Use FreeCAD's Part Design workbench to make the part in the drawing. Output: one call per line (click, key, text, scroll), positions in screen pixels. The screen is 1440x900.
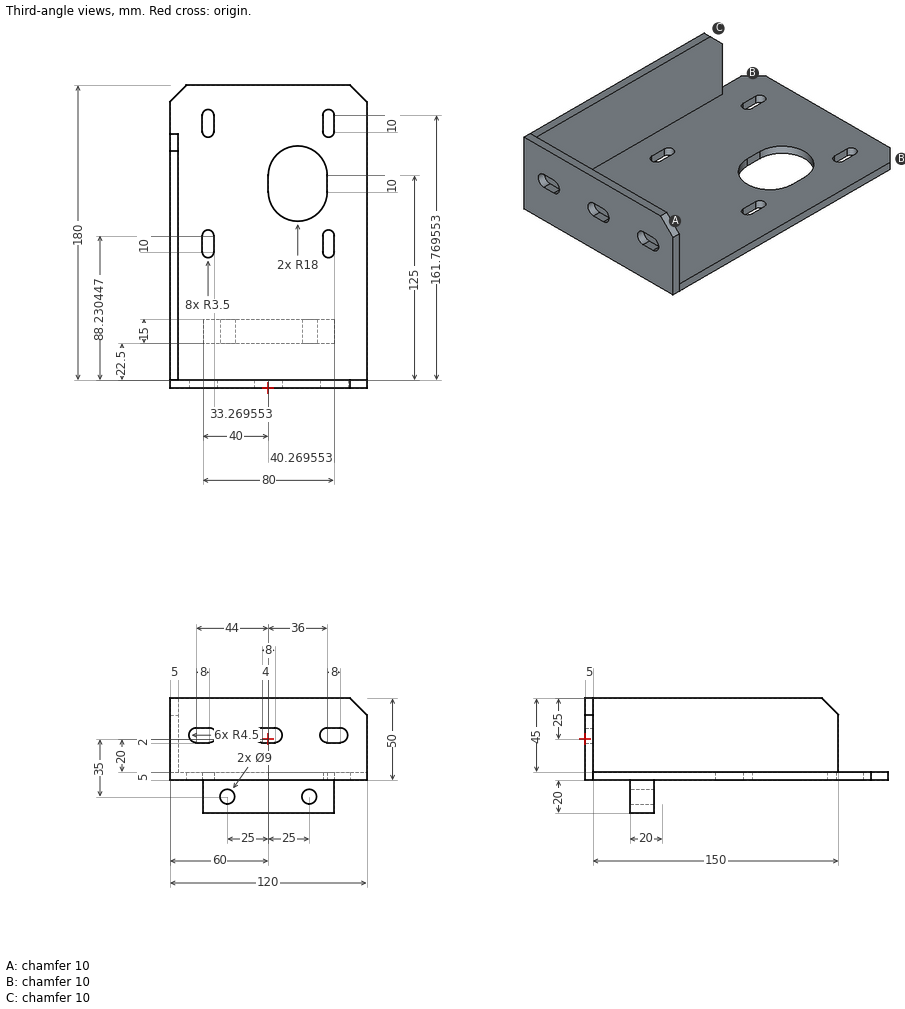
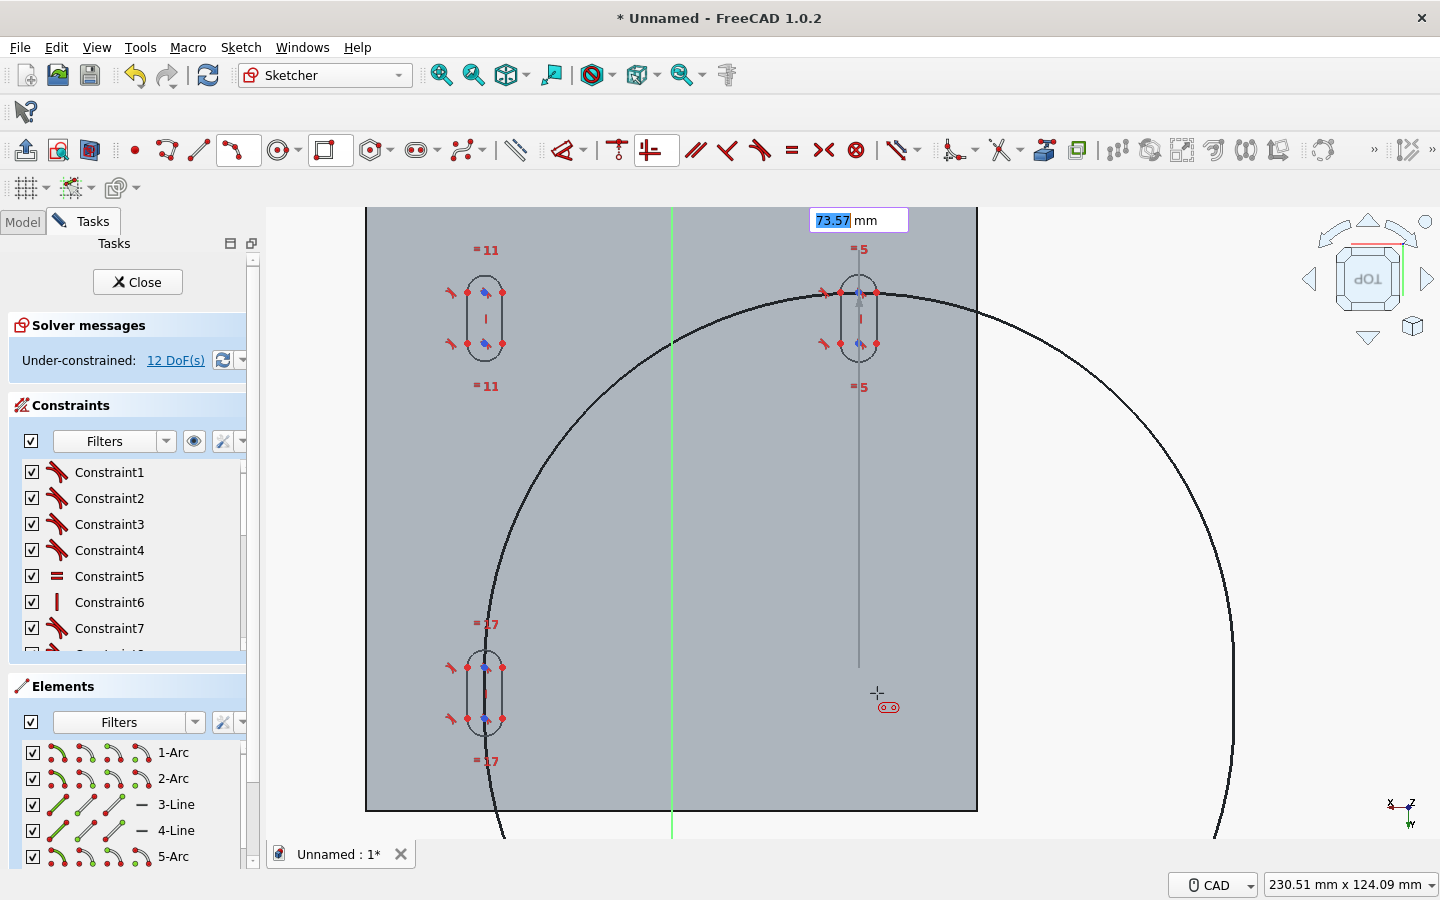
click(877, 692)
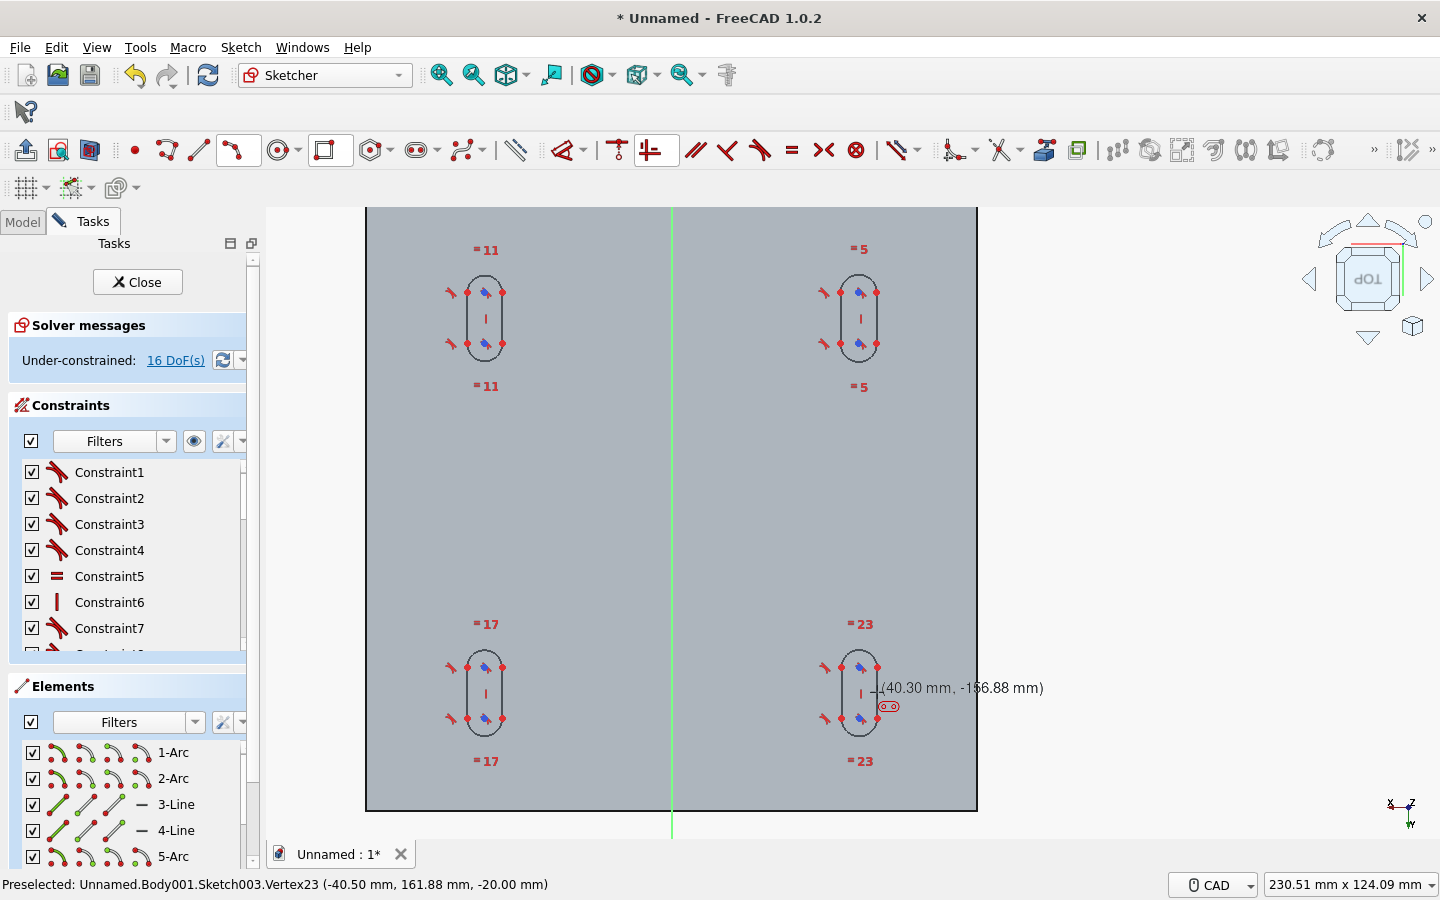
click(580, 531)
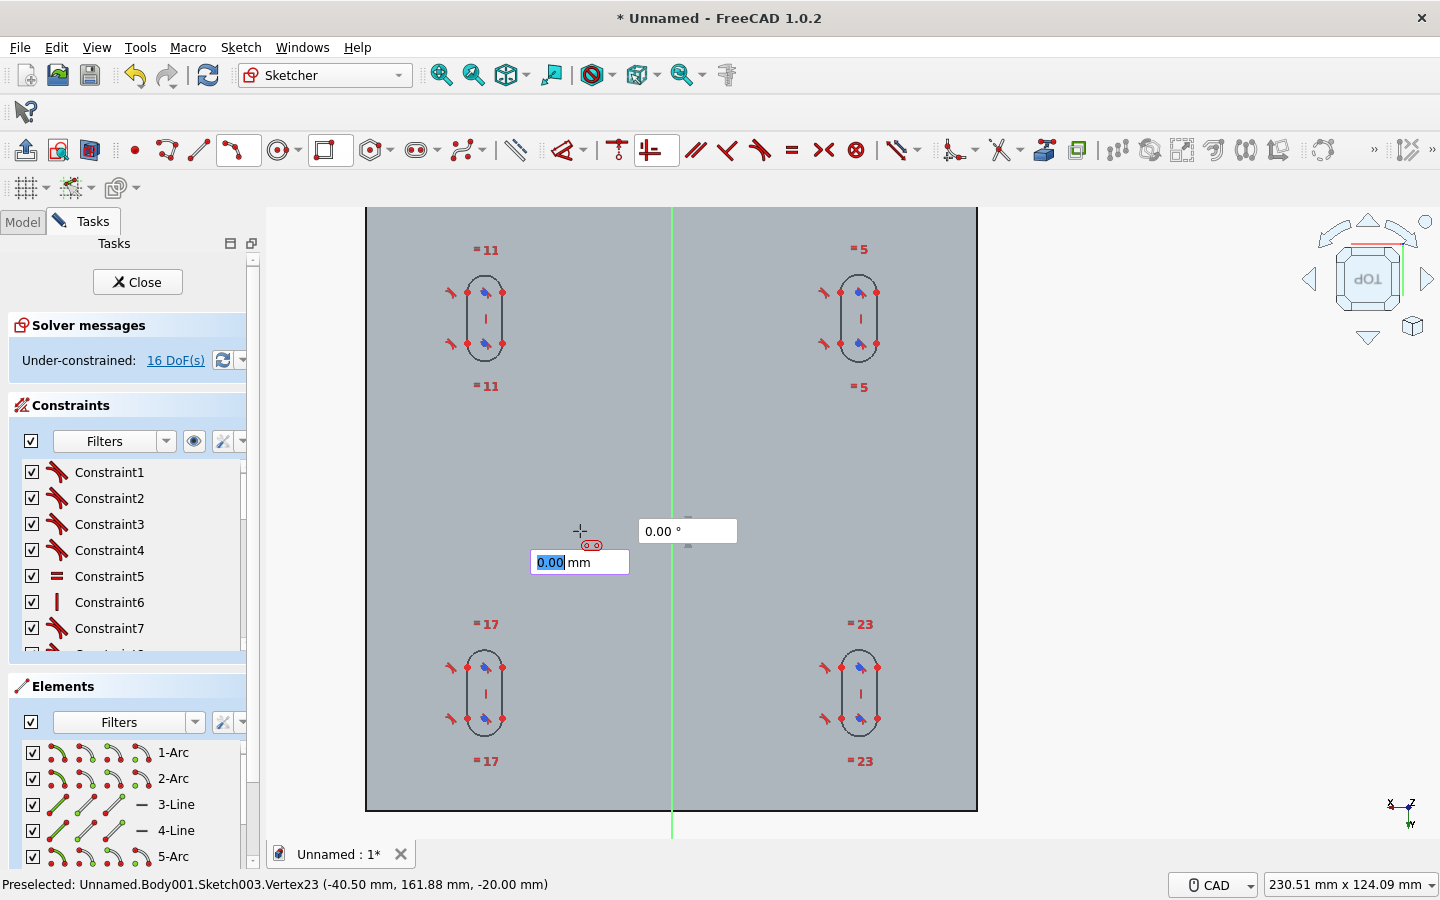
click(580, 480)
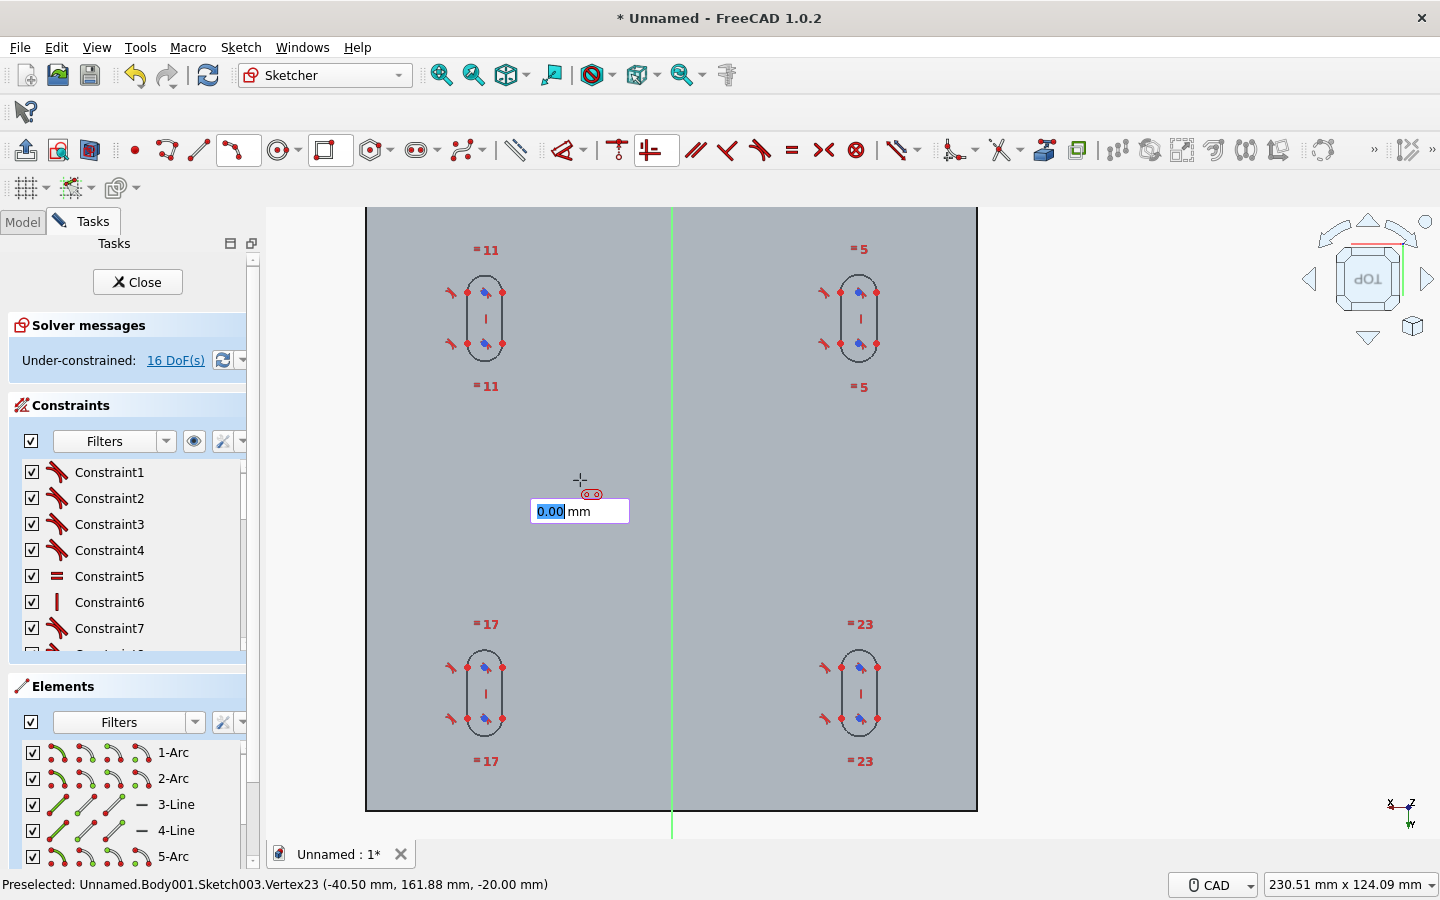
click(488, 505)
key(Escape)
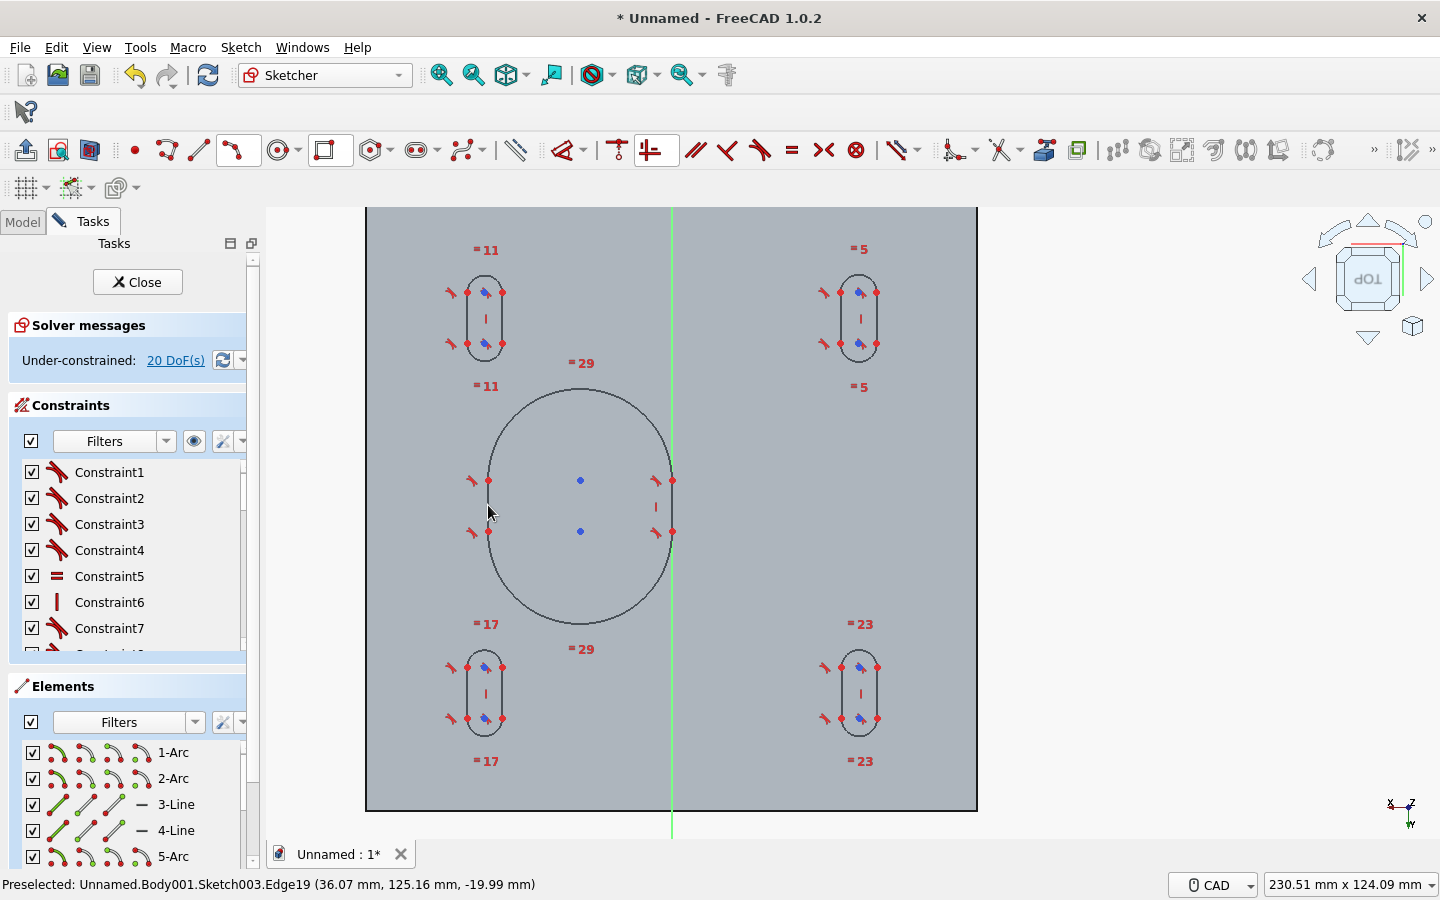
click(848, 359)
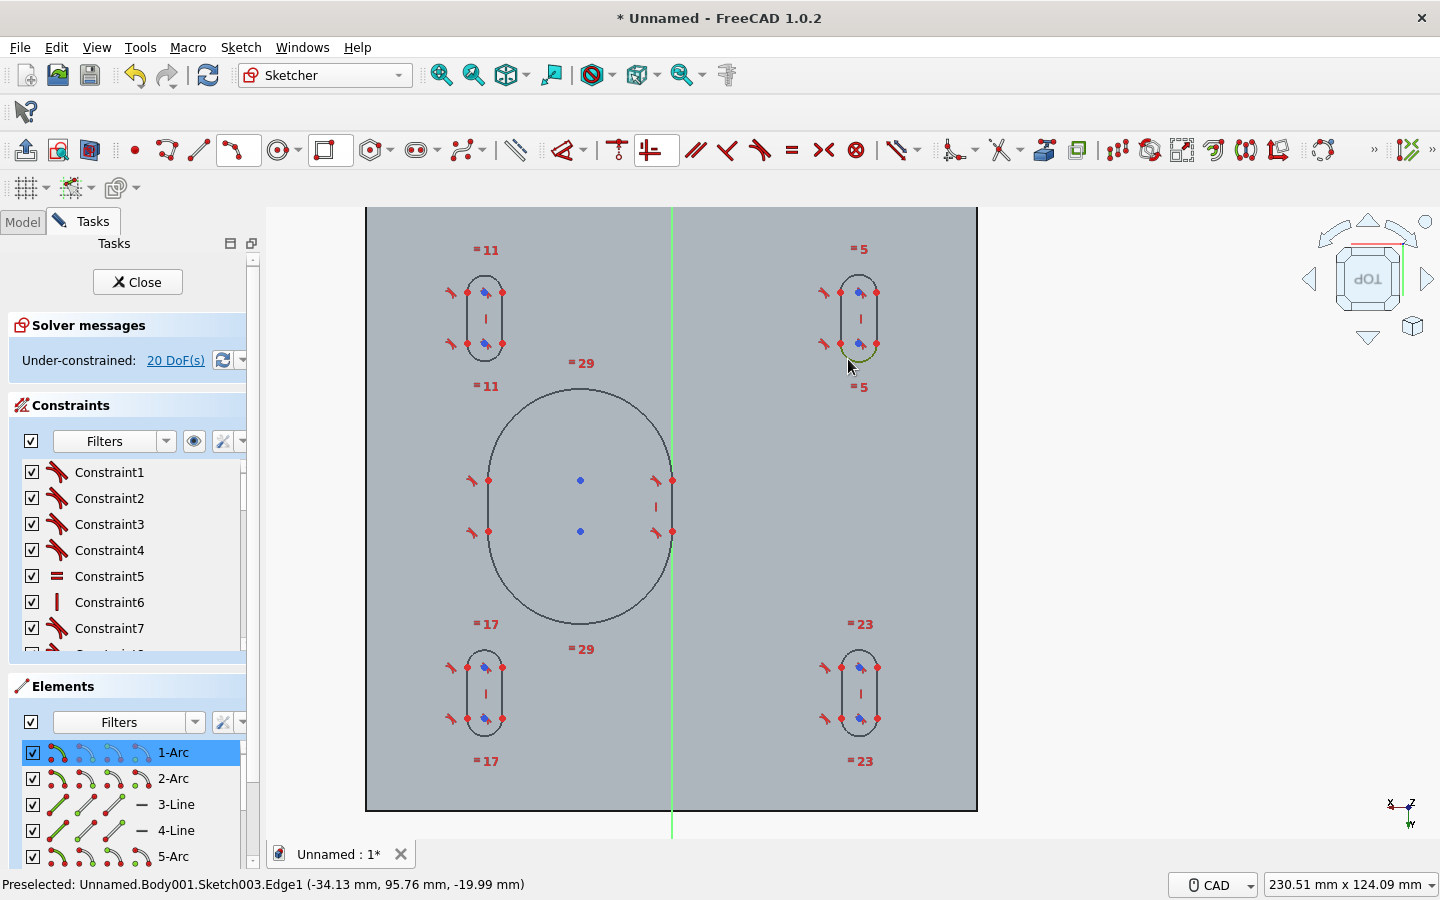
click(474, 358)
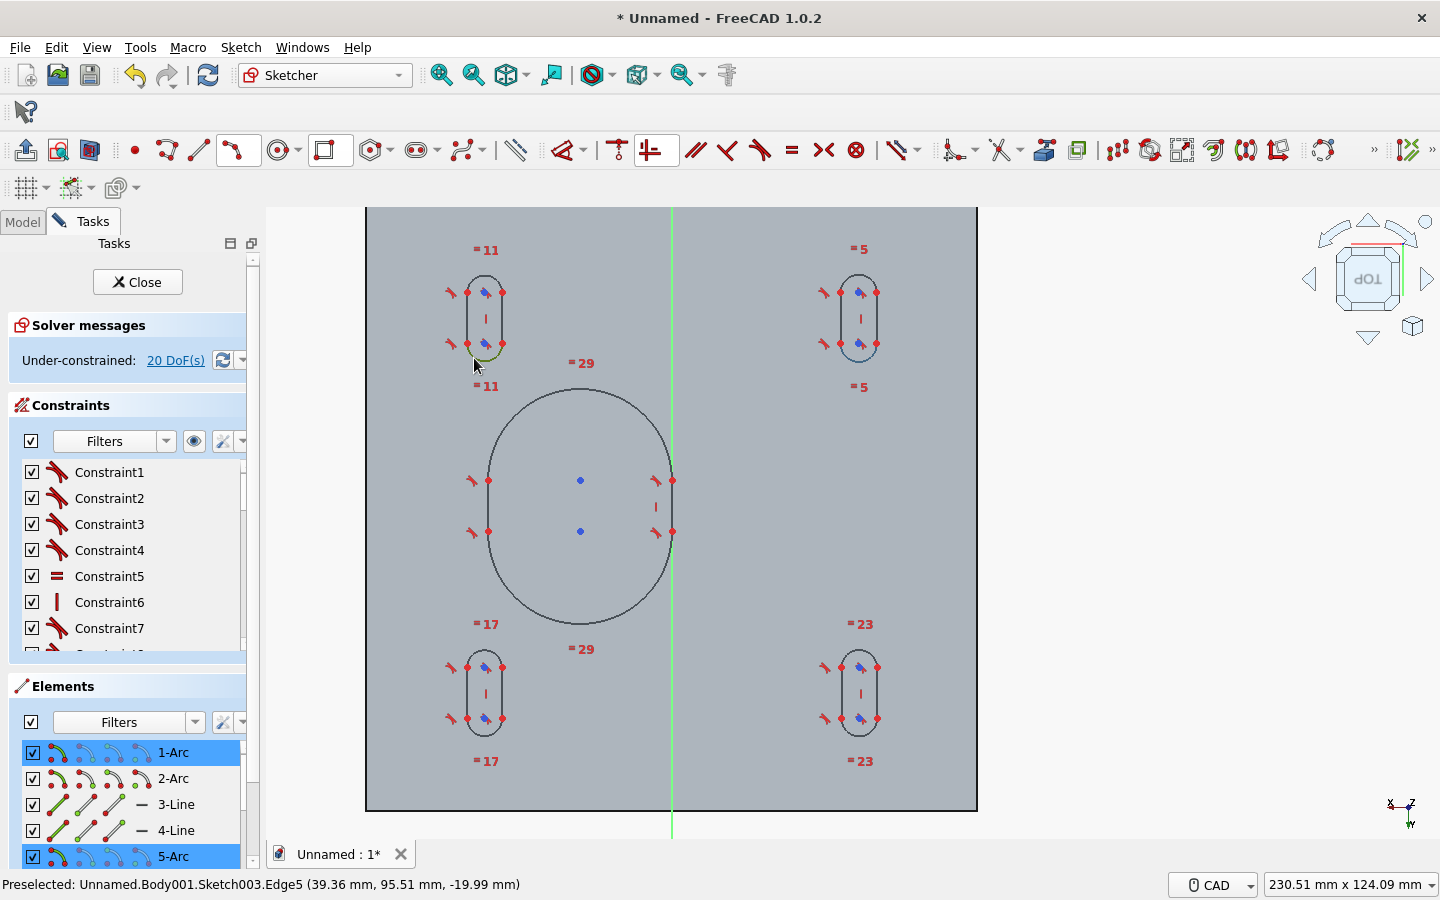
click(474, 733)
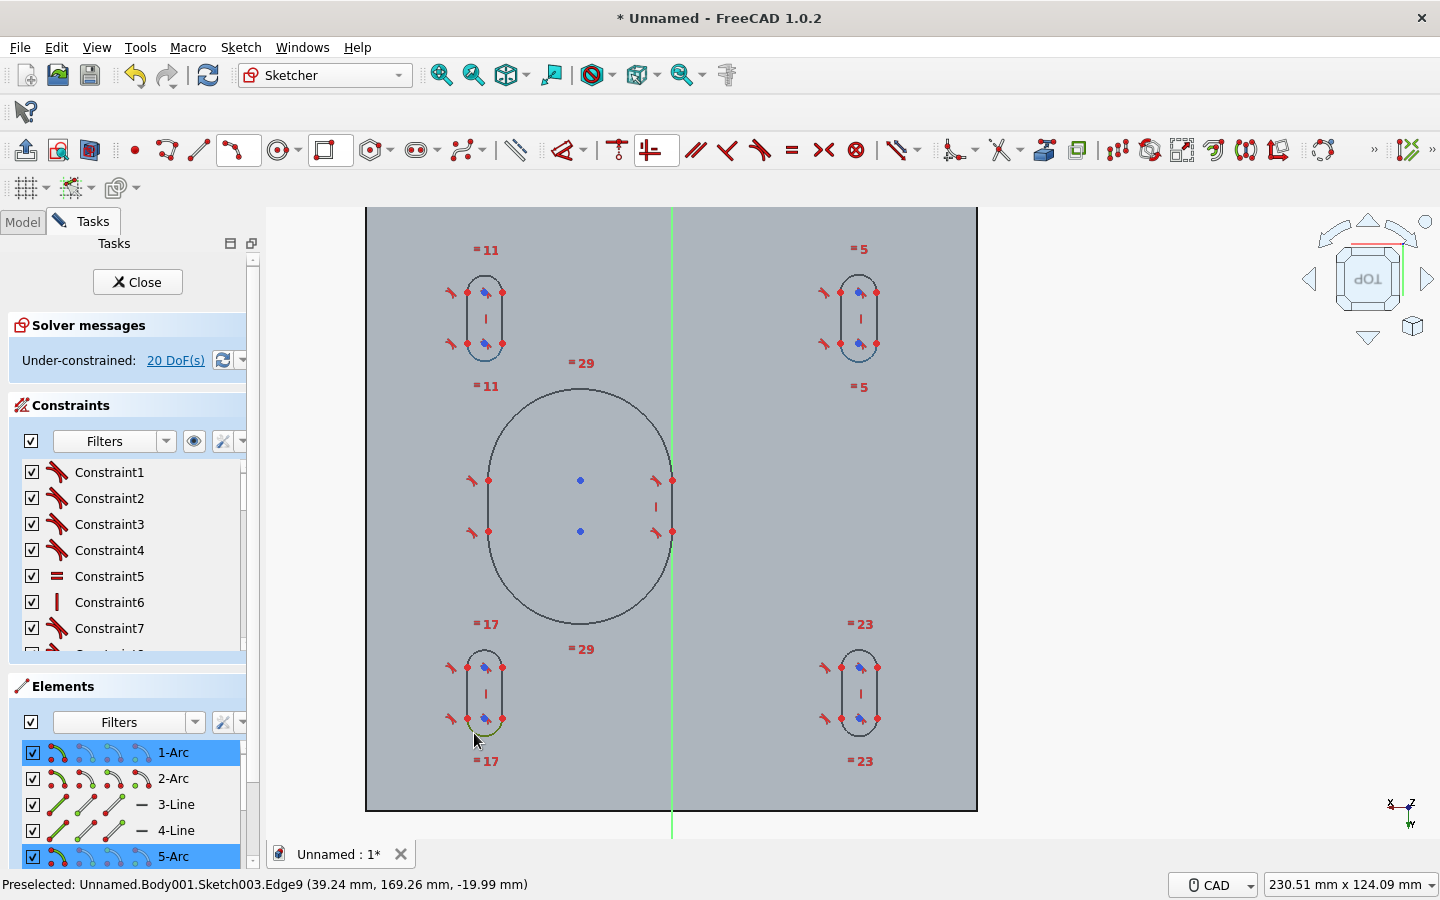
click(849, 733)